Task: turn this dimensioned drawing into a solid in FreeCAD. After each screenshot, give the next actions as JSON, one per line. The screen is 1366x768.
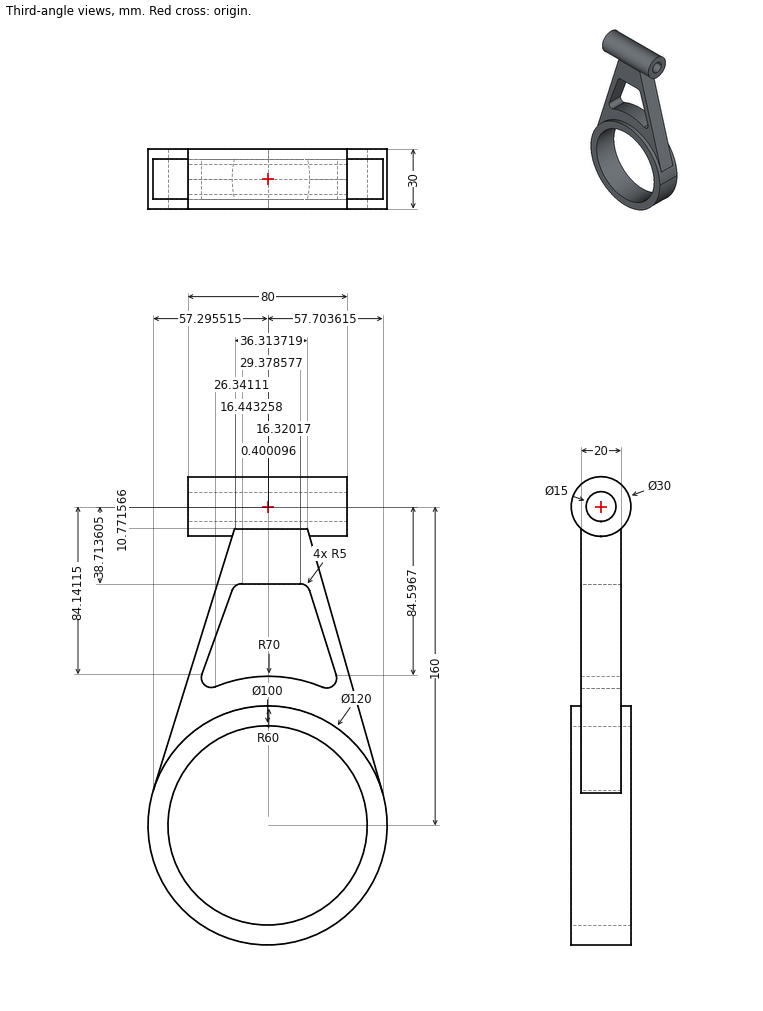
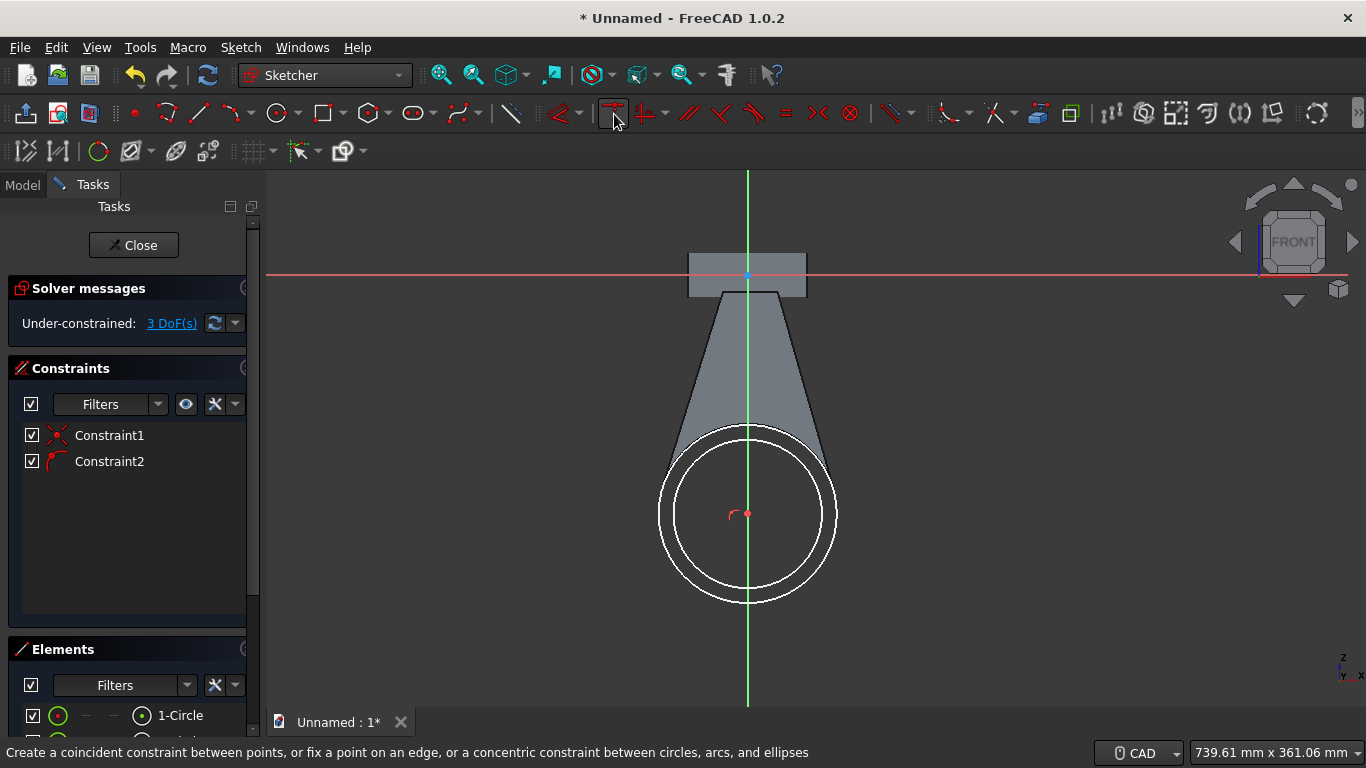
{"action": "left_click", "coordinate": [811, 451]}
{"action": "left_click", "coordinate": [834, 428]}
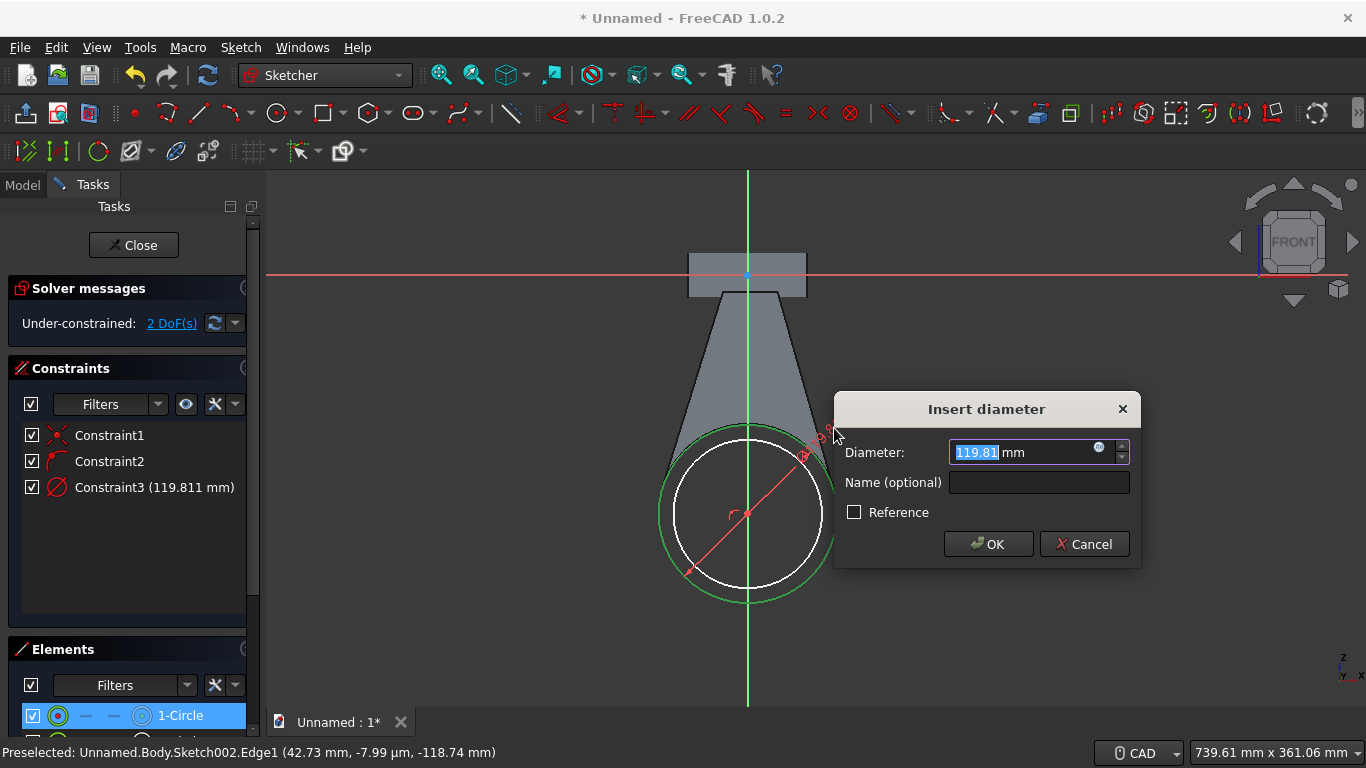
{"action": "type", "text": "120"}
{"action": "key", "text": "Return"}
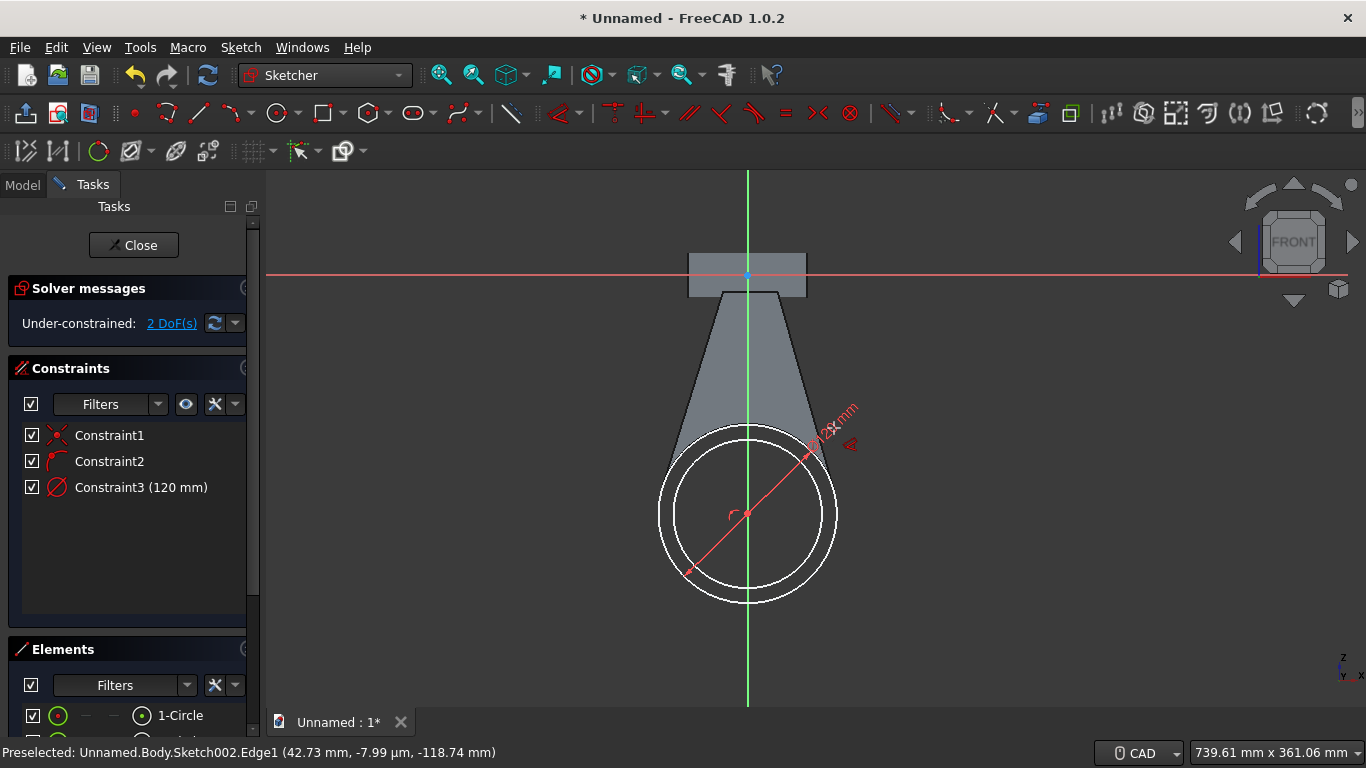
{"action": "left_click", "coordinate": [800, 461]}
{"action": "left_click", "coordinate": [850, 483]}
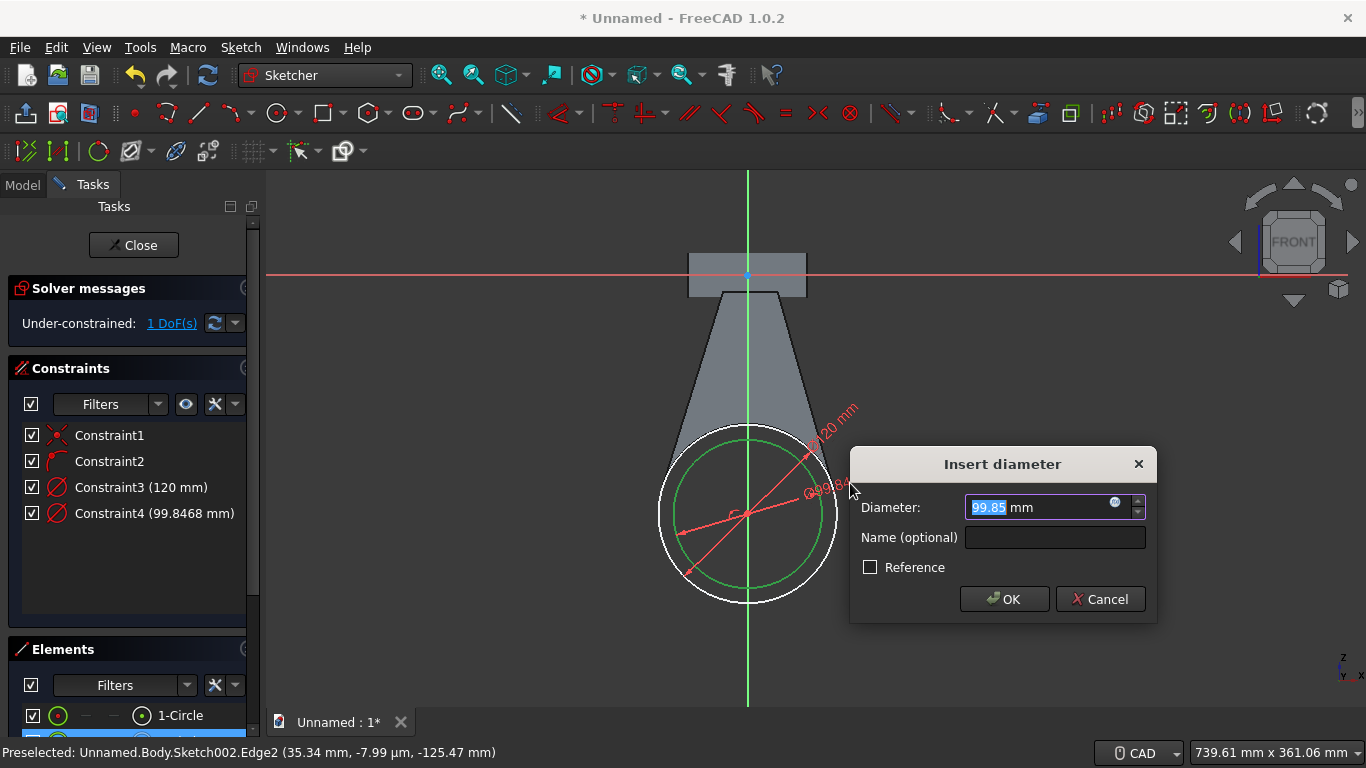
{"action": "type", "text": "100"}
{"action": "key", "text": "Return"}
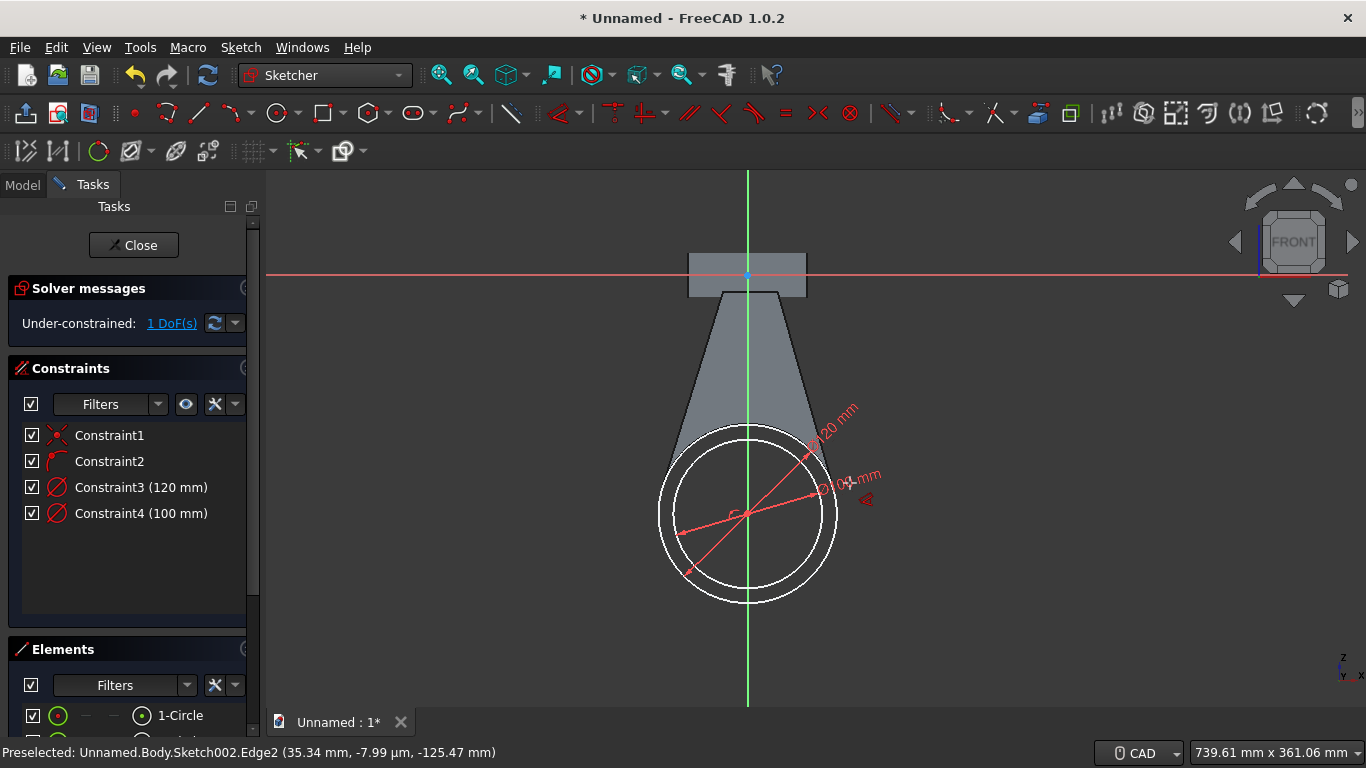
{"action": "left_click", "coordinate": [748, 514]}
{"action": "left_click", "coordinate": [782, 395]}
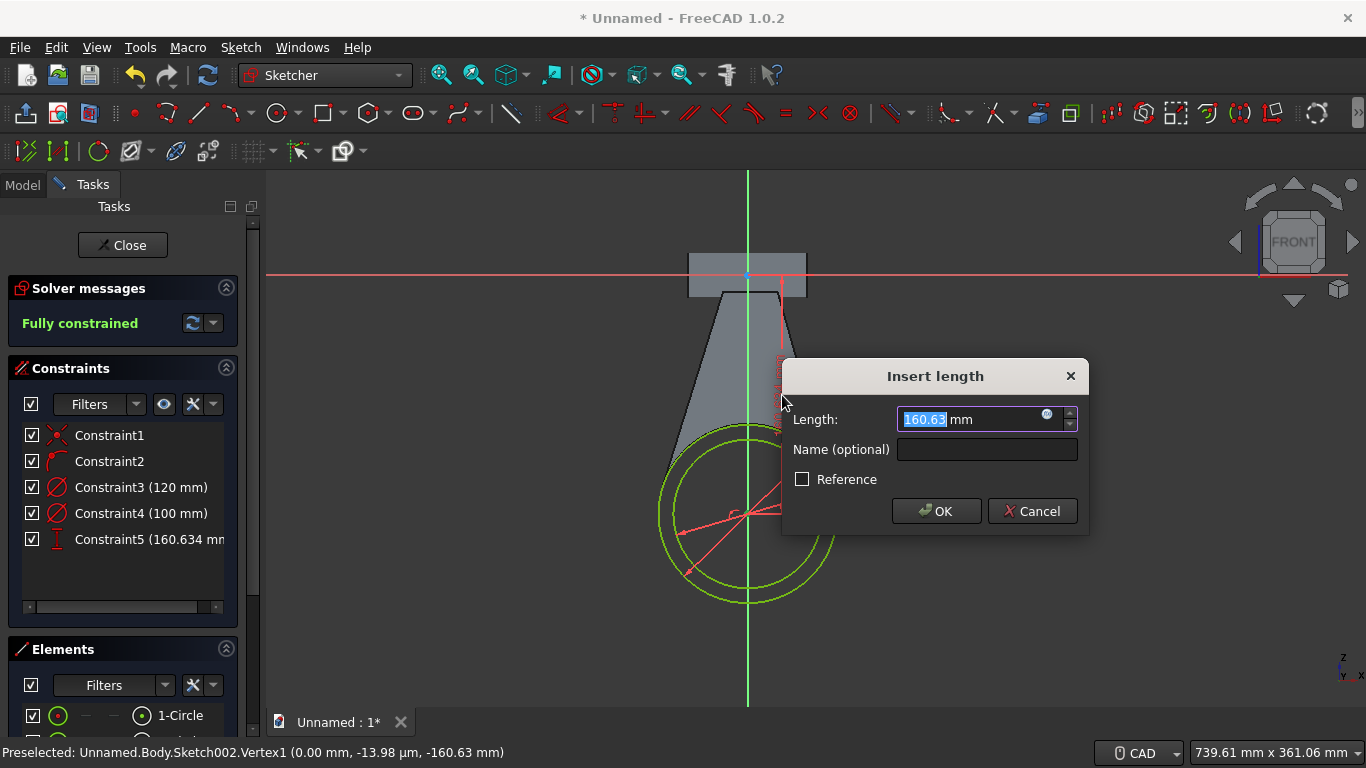
{"action": "type", "text": "160"}
{"action": "key", "text": "Return"}
{"action": "key", "text": "Escape"}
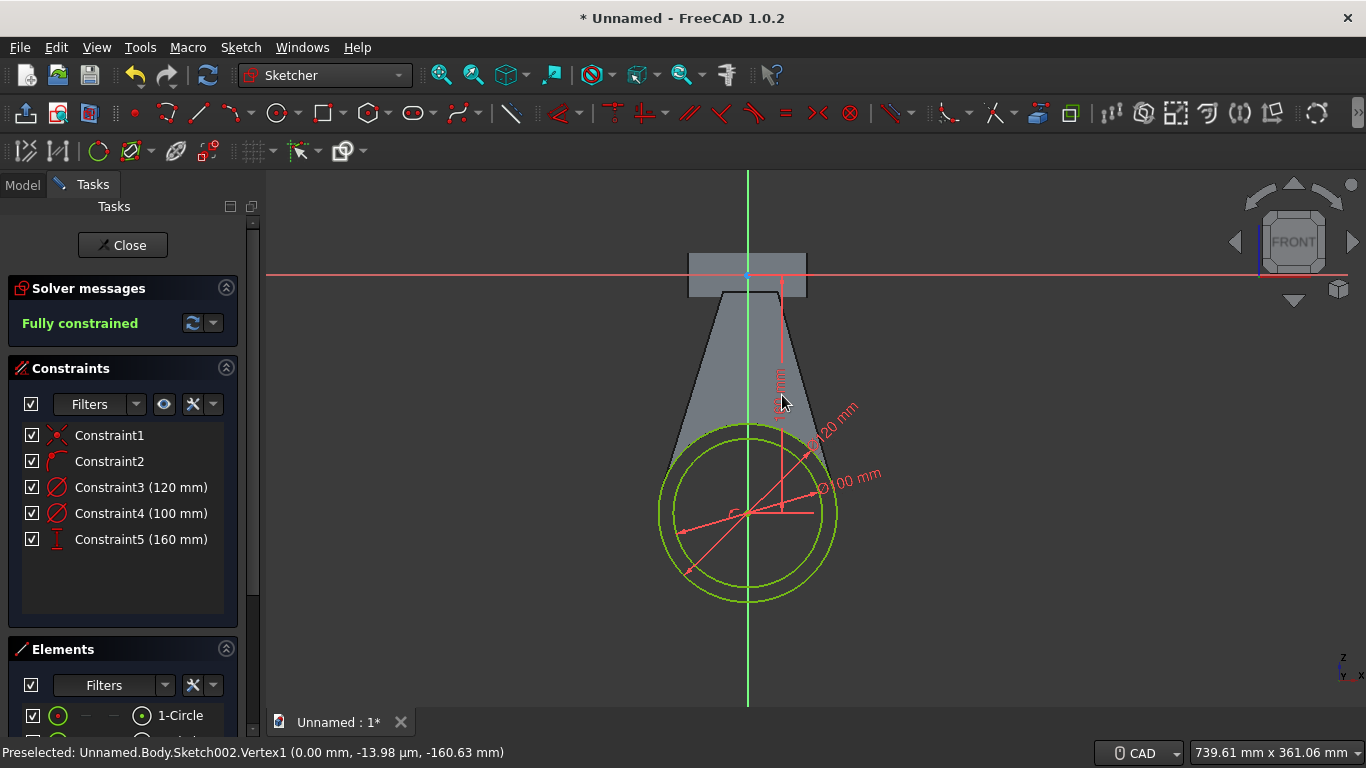
{"action": "left_click", "coordinate": [123, 245]}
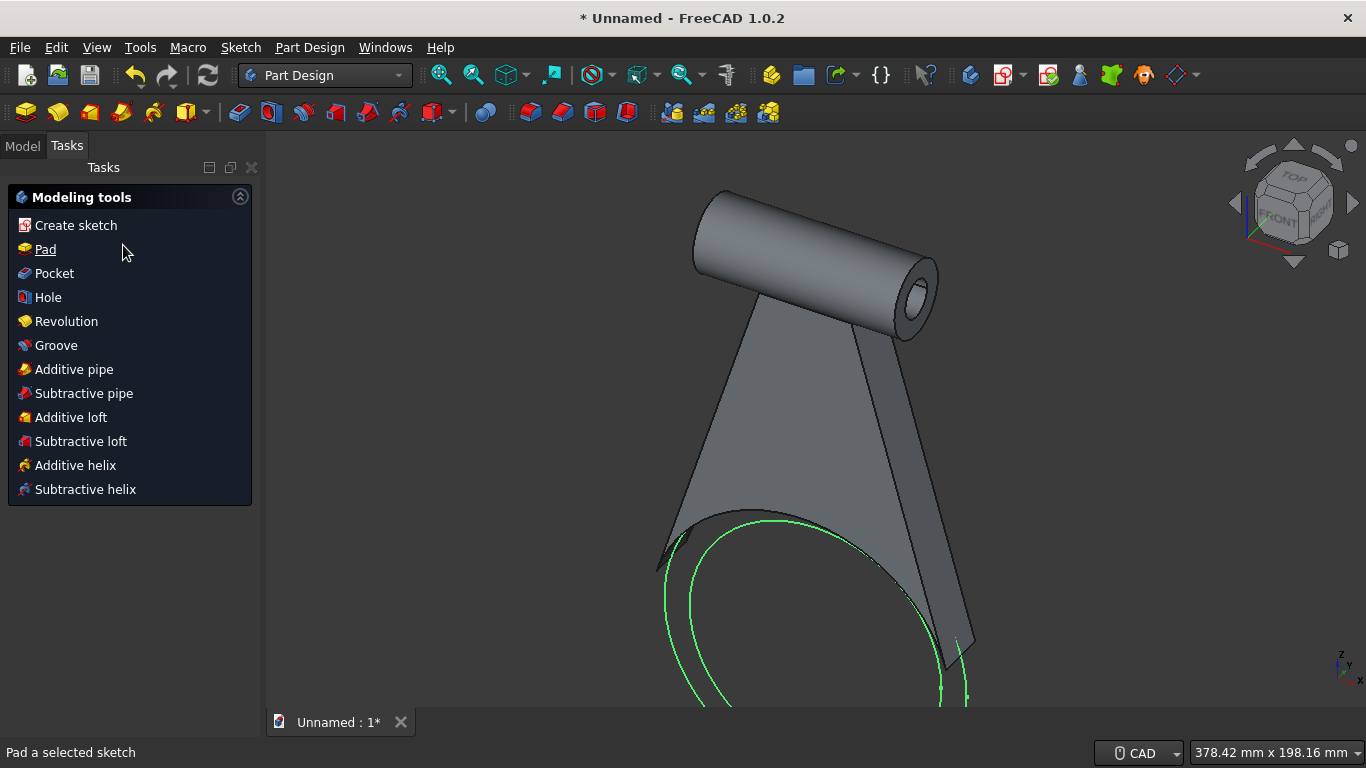
{"action": "left_click", "coordinate": [26, 112]}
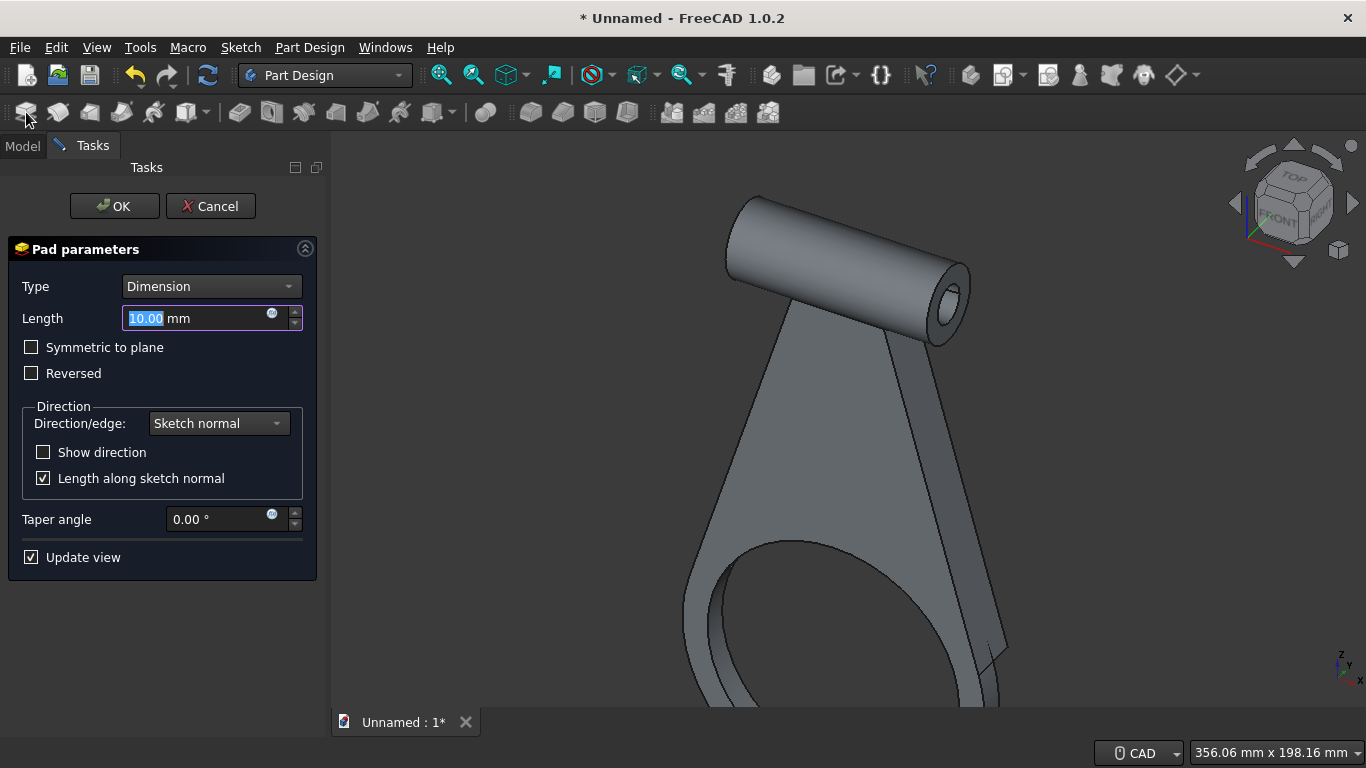
{"action": "type", "text": "30"}
{"action": "key", "text": "Tab"}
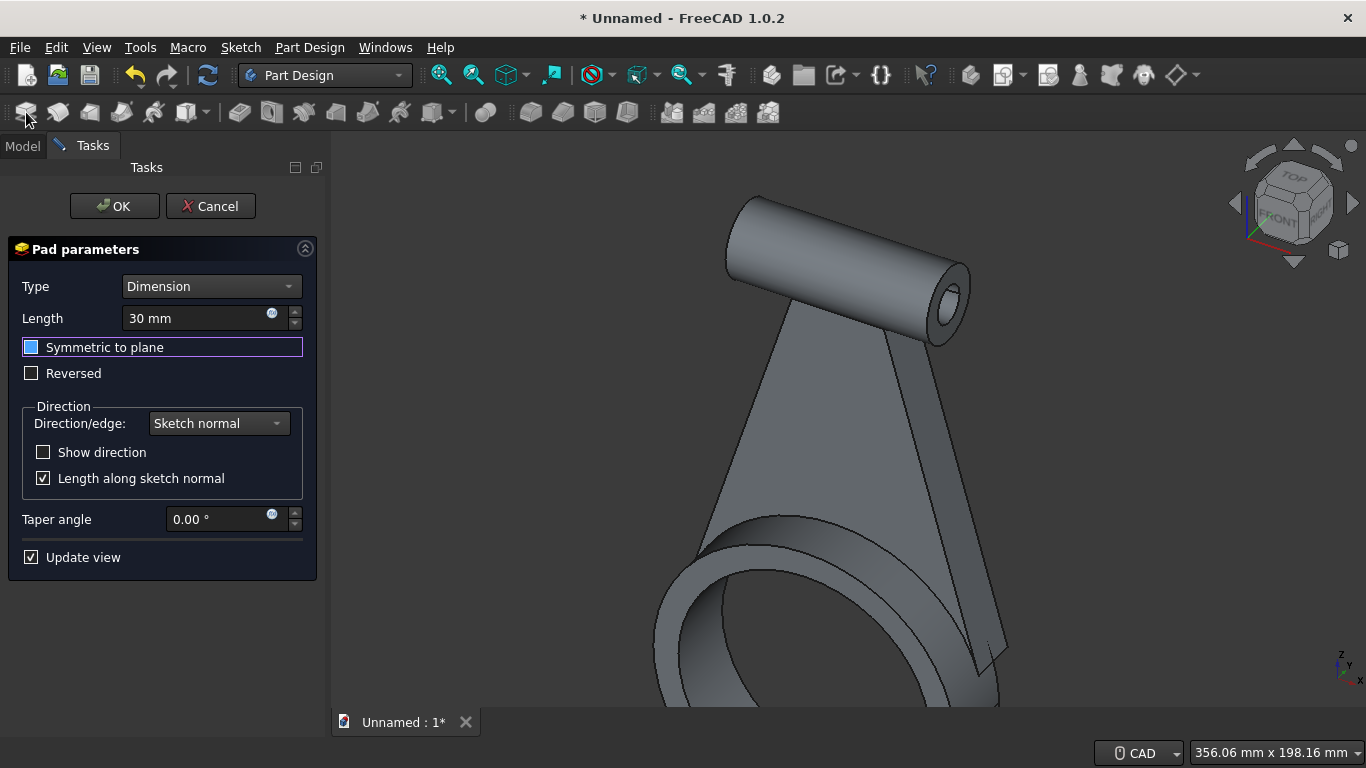
{"action": "left_click", "coordinate": [30, 347]}